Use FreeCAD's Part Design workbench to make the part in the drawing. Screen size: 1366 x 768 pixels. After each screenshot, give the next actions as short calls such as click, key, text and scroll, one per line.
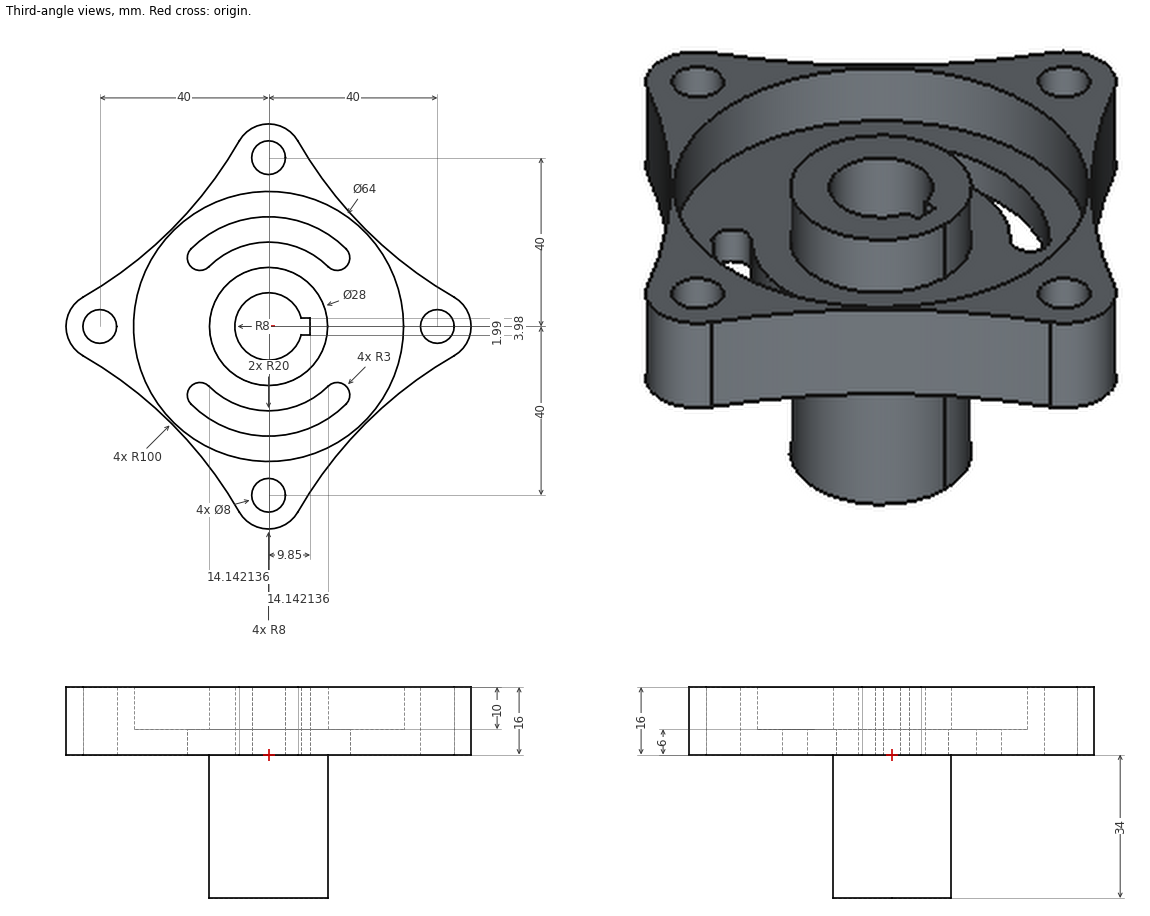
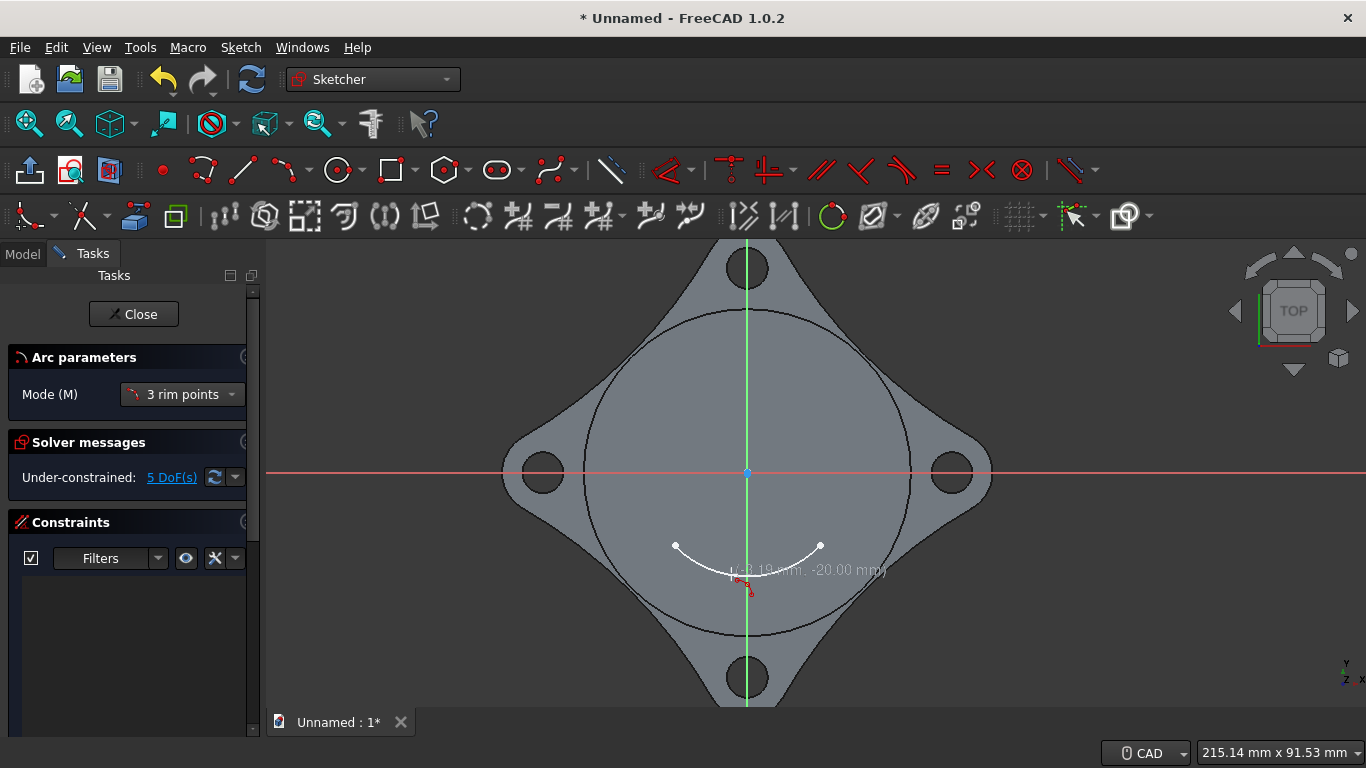
click(675, 546)
click(653, 567)
click(653, 545)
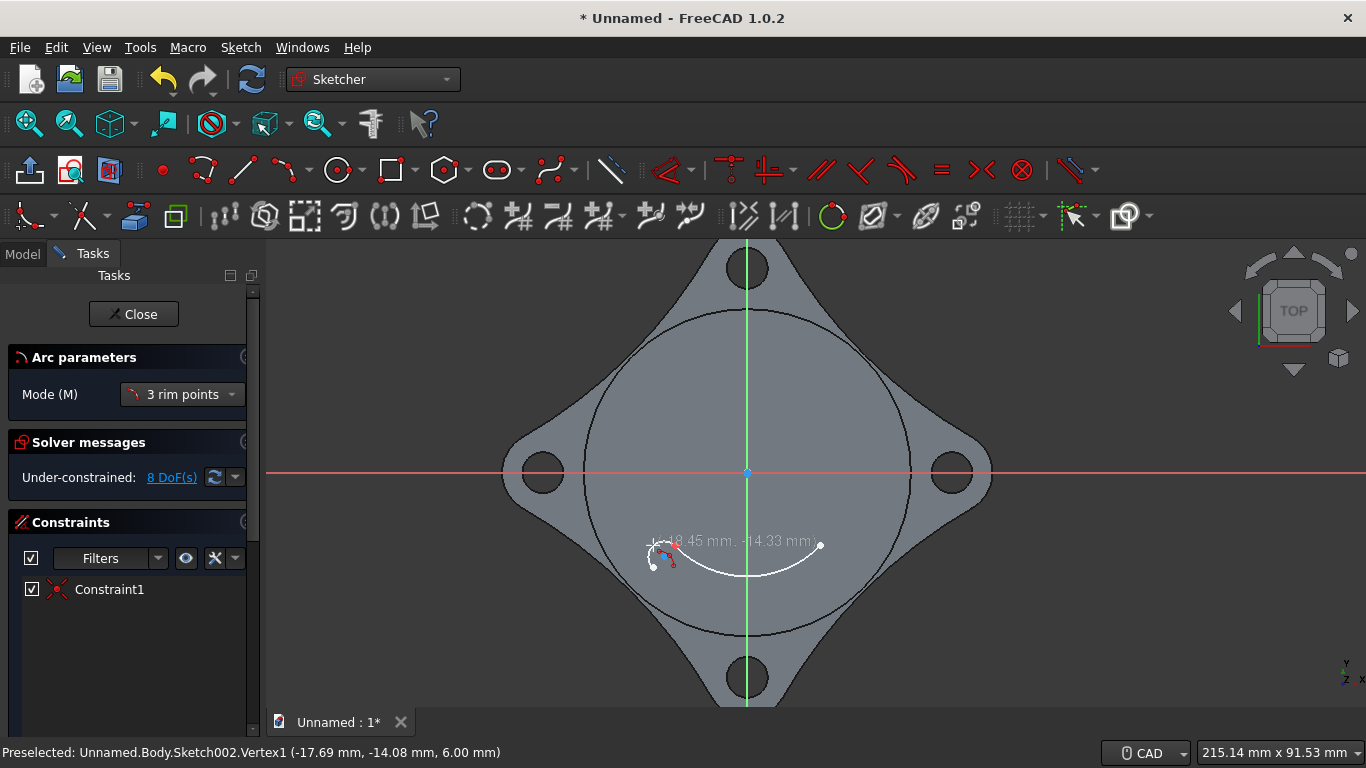
click(653, 568)
click(841, 567)
click(727, 604)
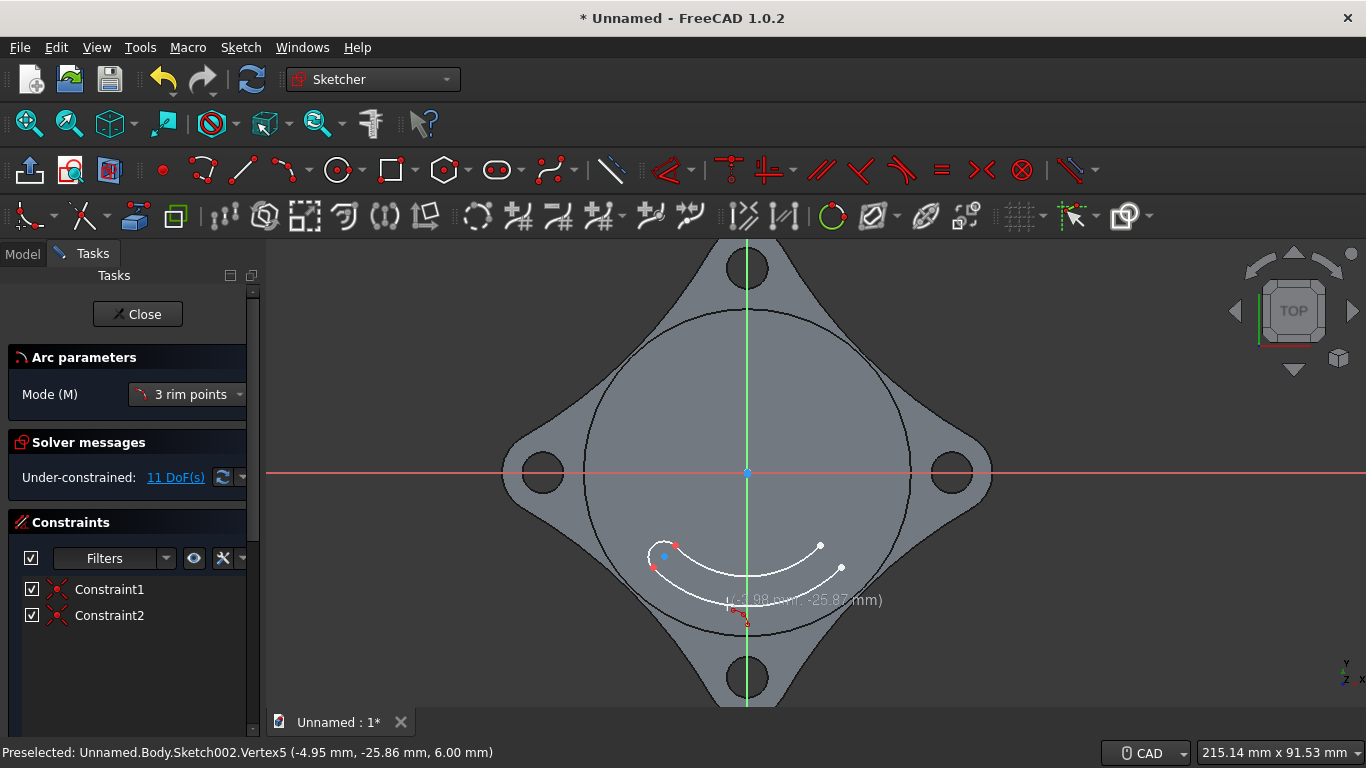
click(841, 568)
click(820, 546)
click(841, 545)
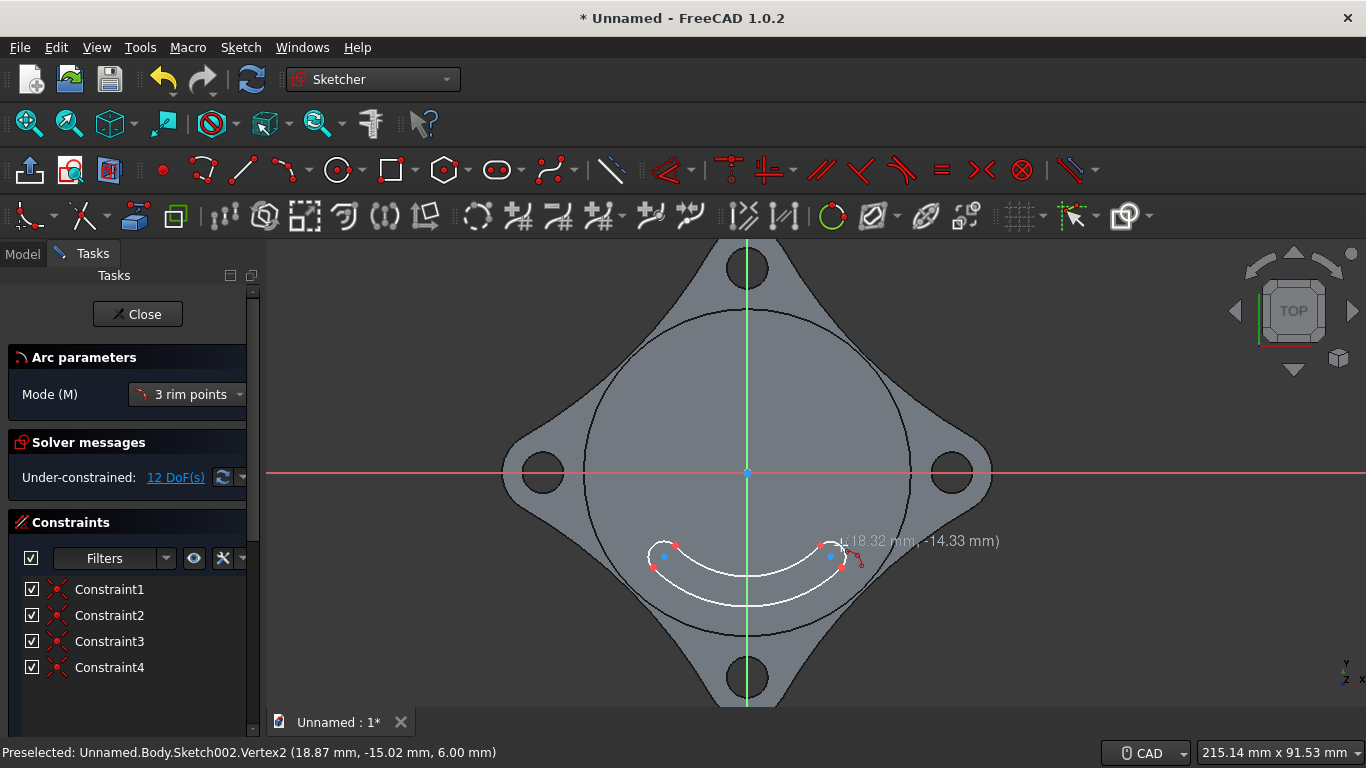
click(675, 400)
click(820, 400)
click(763, 372)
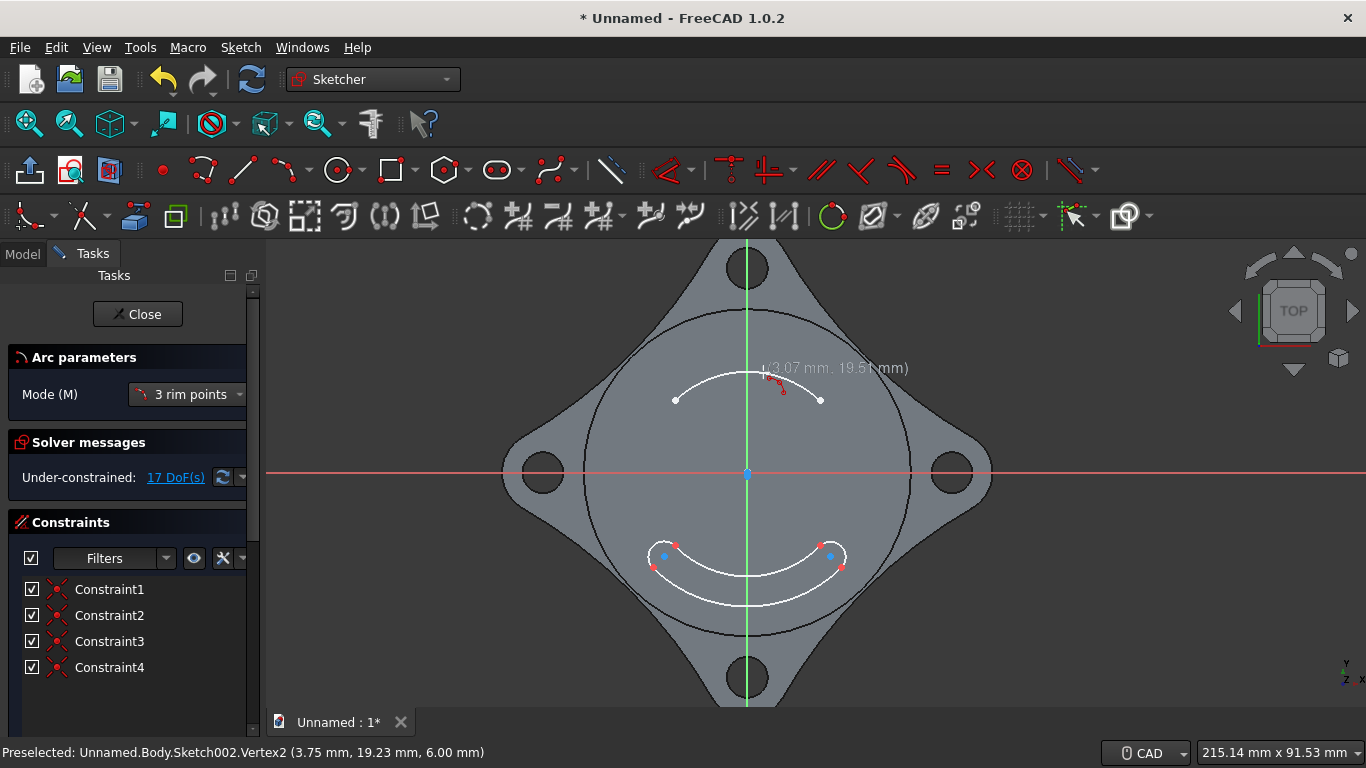
click(820, 401)
click(841, 379)
click(841, 400)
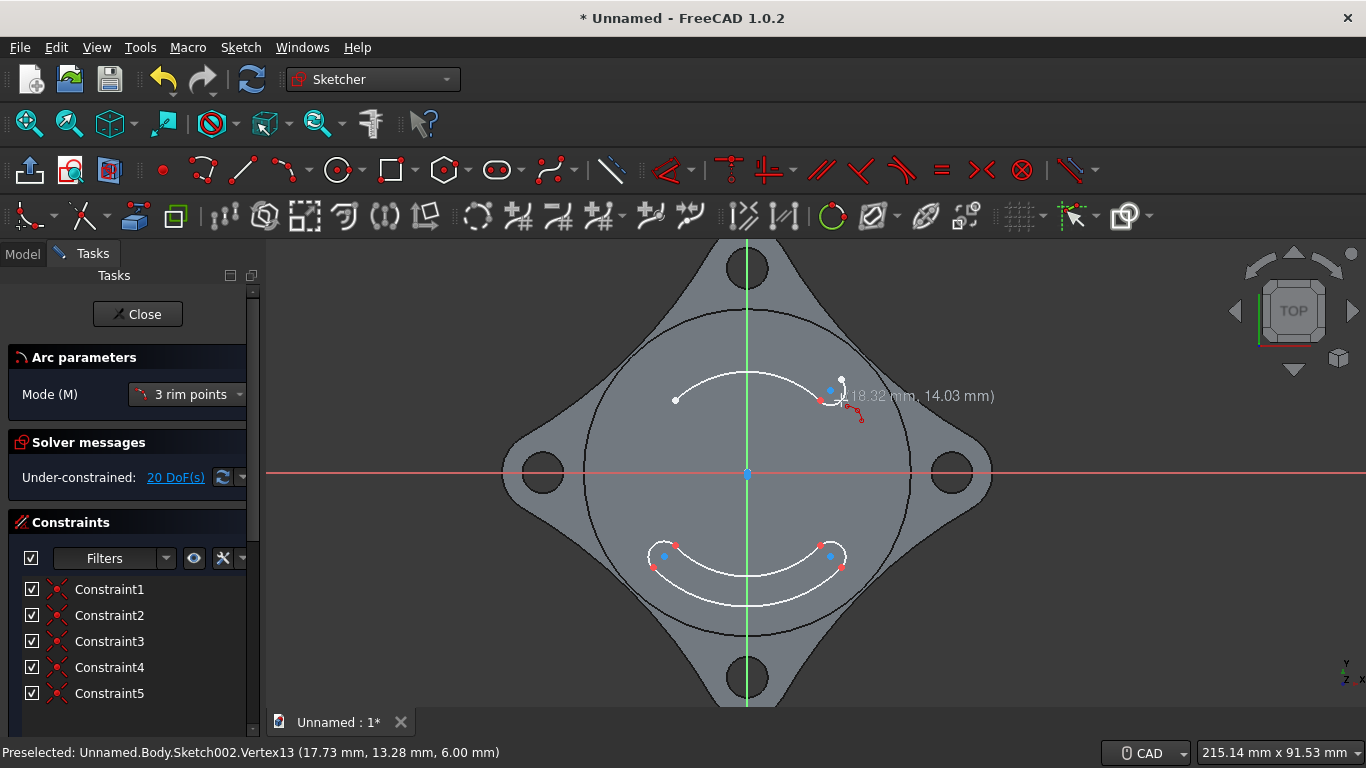
click(841, 380)
click(653, 379)
click(768, 341)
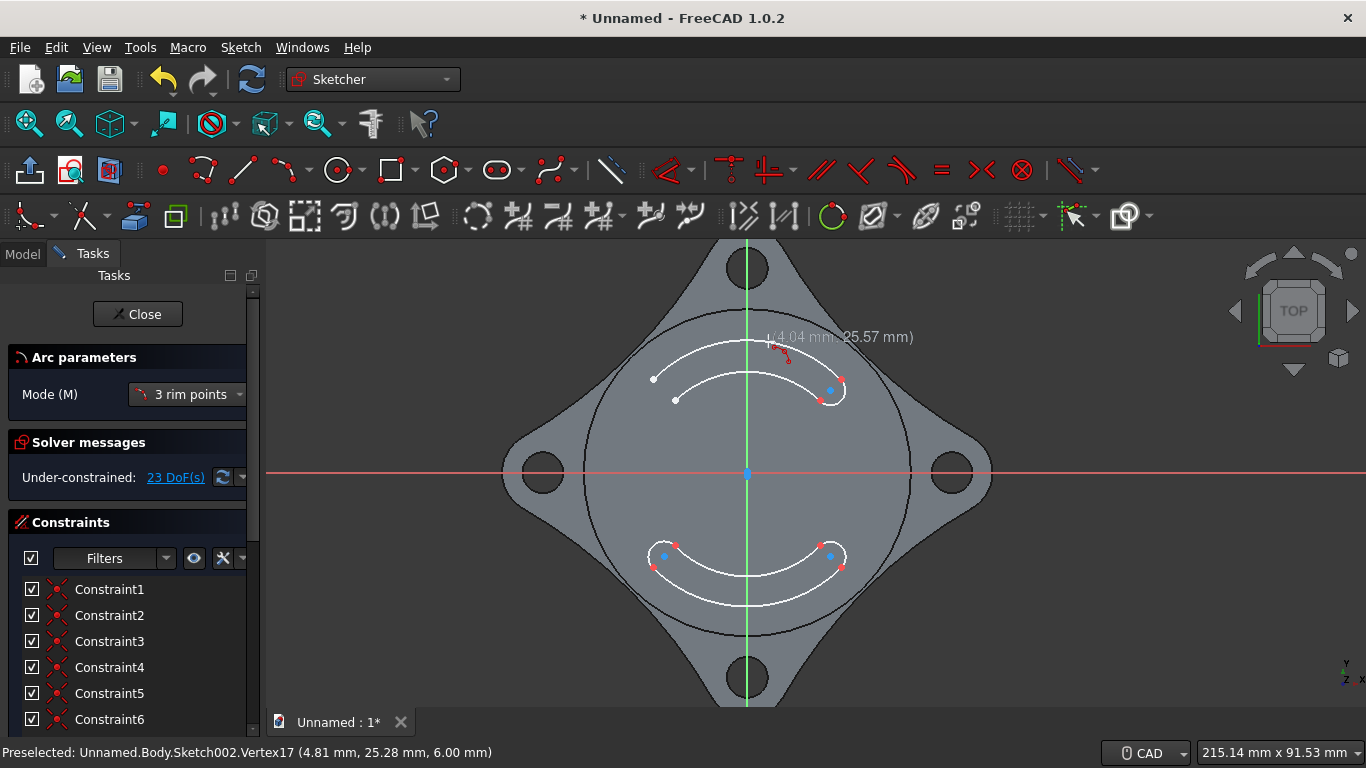
click(653, 380)
click(675, 401)
click(653, 400)
key(Escape)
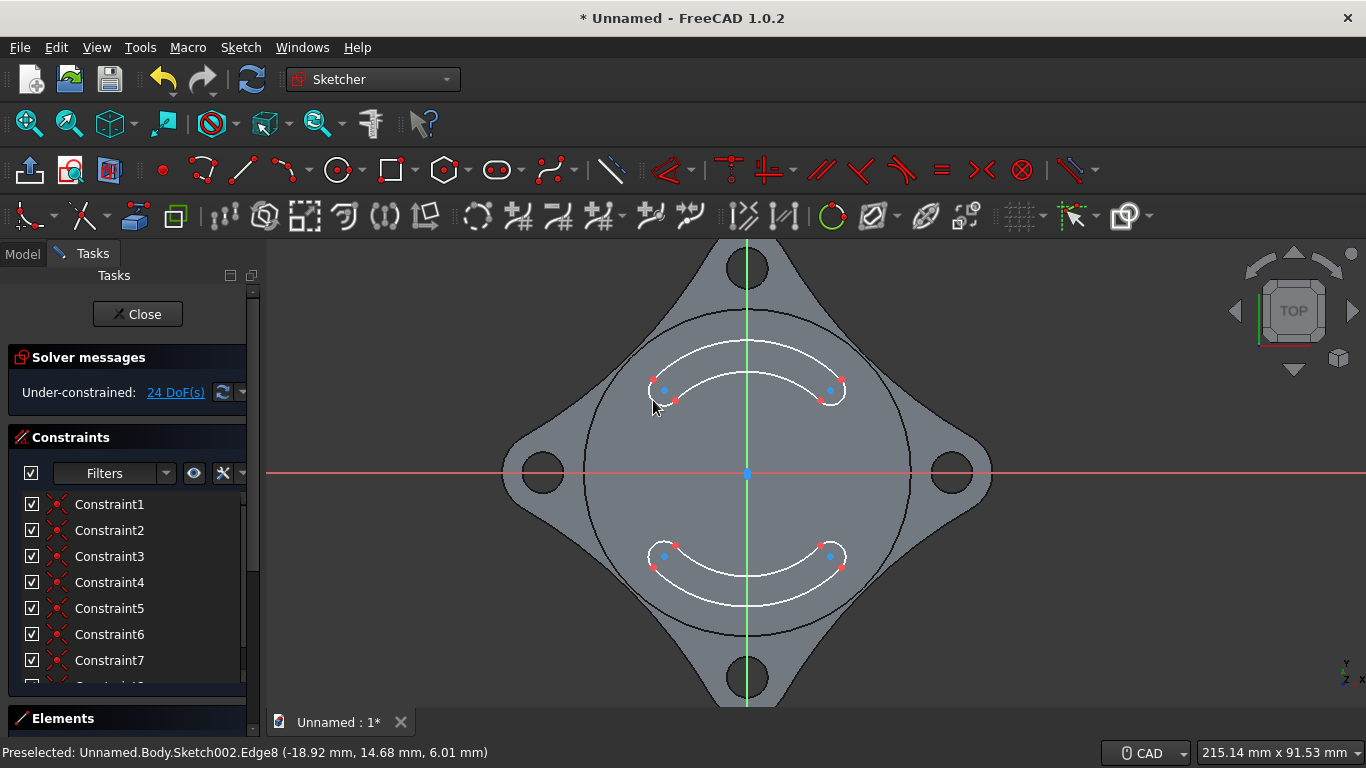
click(716, 571)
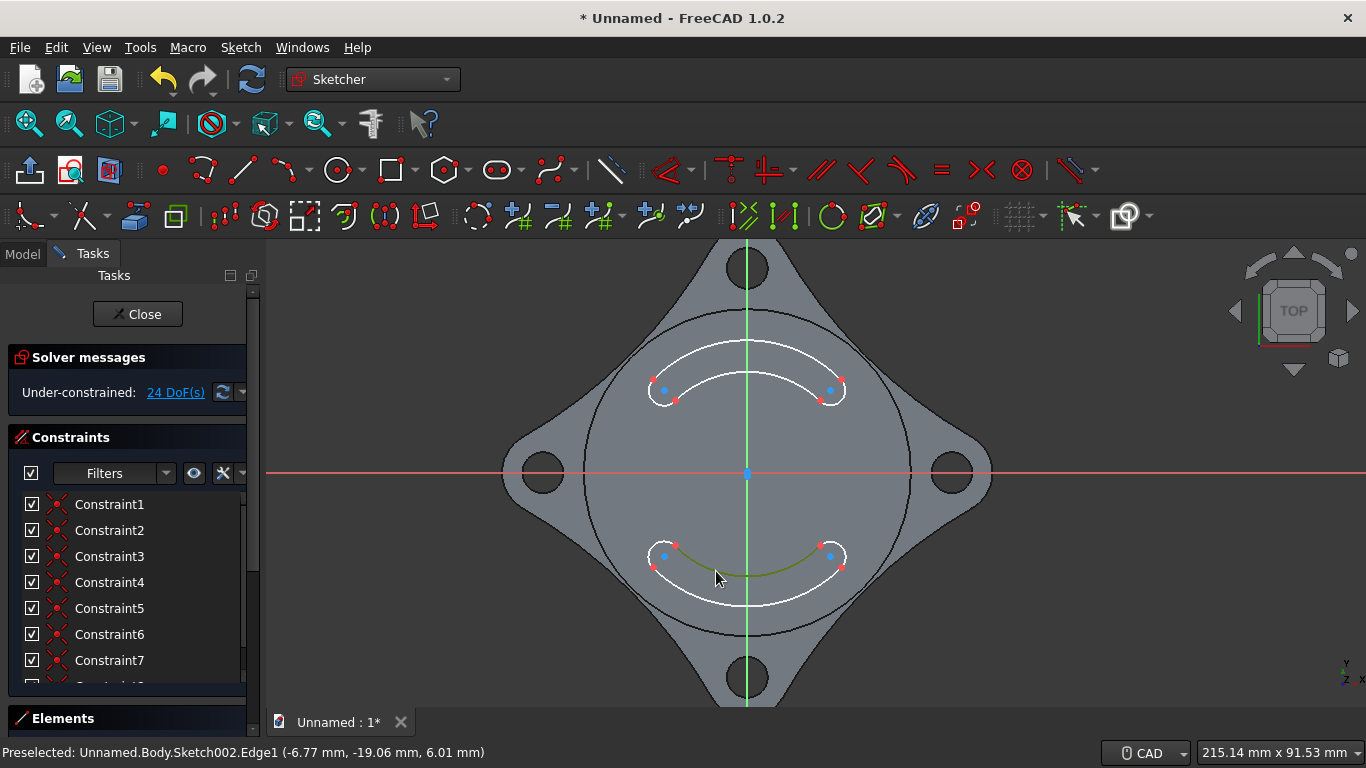
click(662, 542)